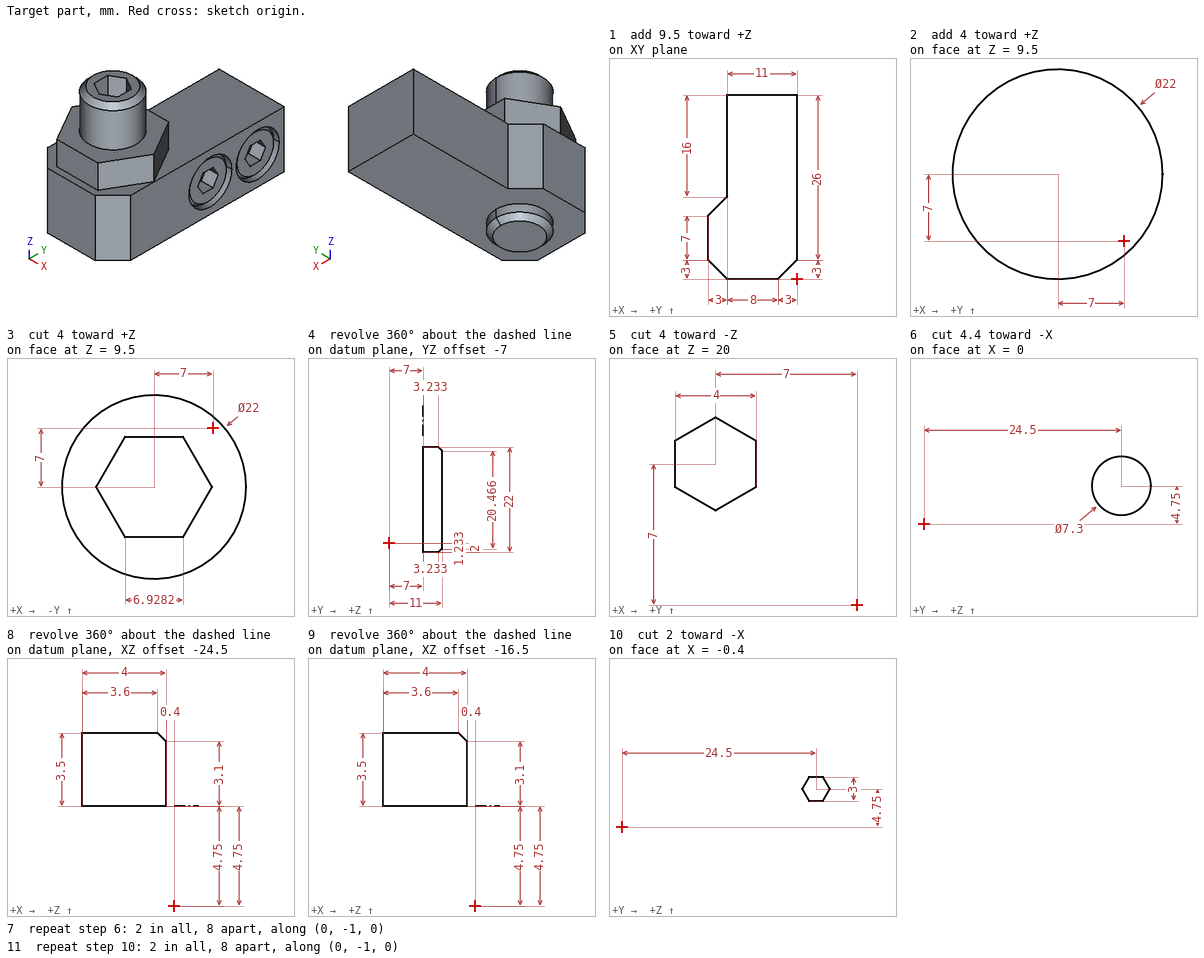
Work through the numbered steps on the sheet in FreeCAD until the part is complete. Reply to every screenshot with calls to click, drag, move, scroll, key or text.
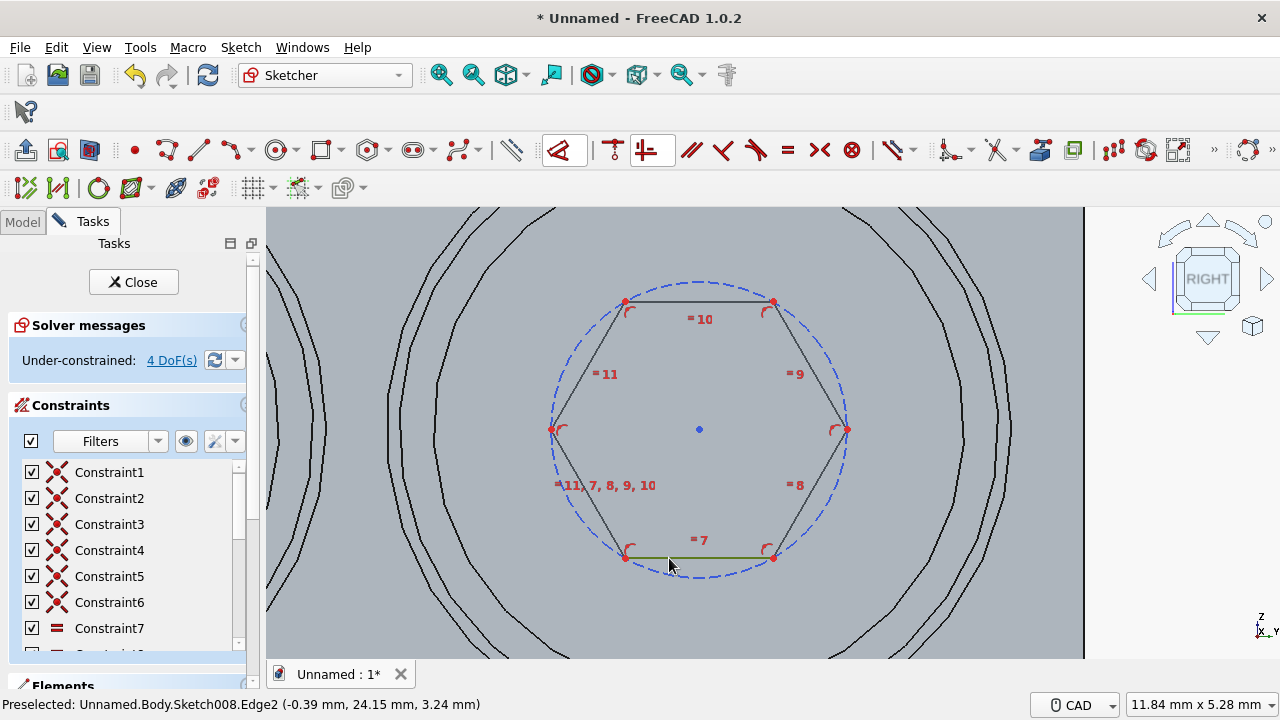
click(670, 150)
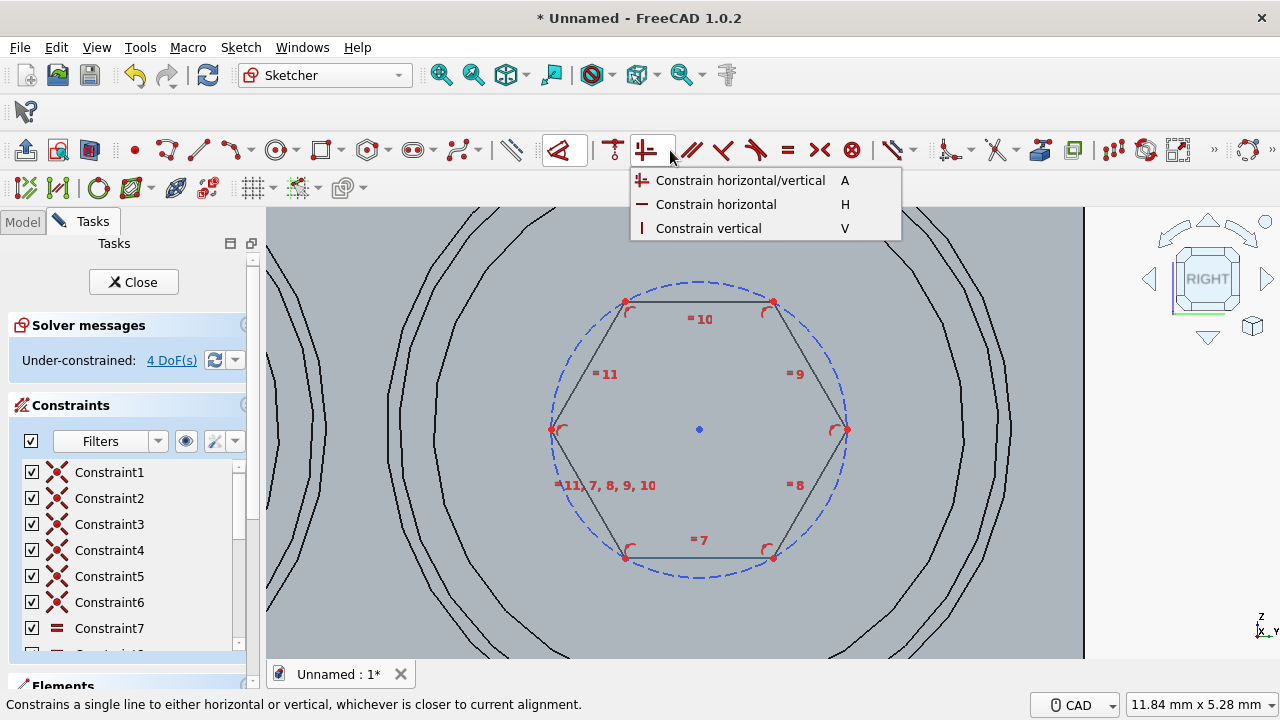
click(766, 204)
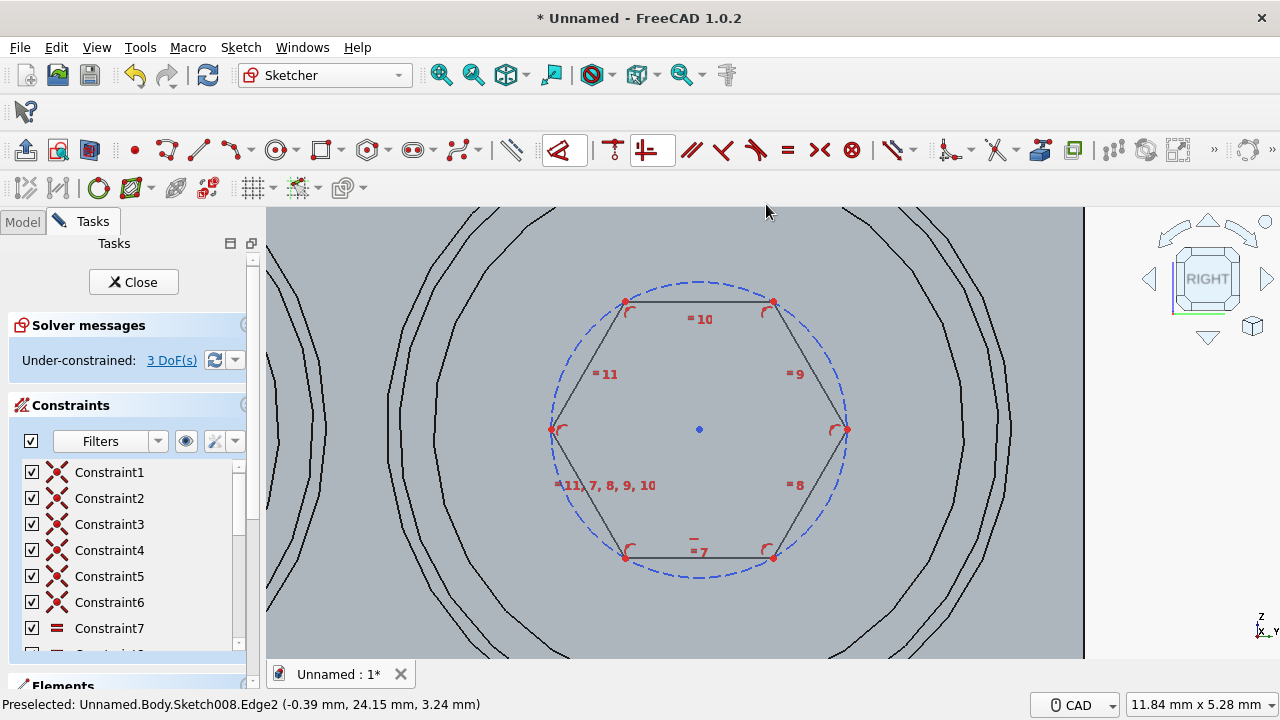
click(625, 558)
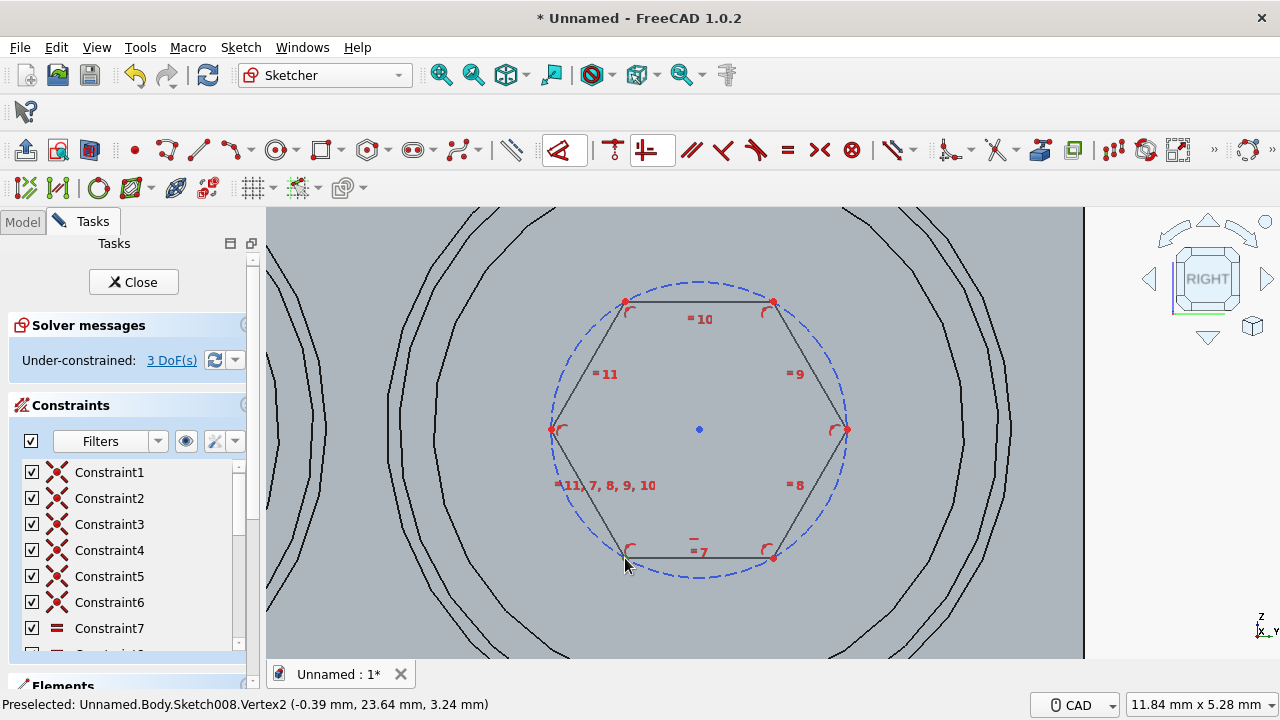
click(773, 302)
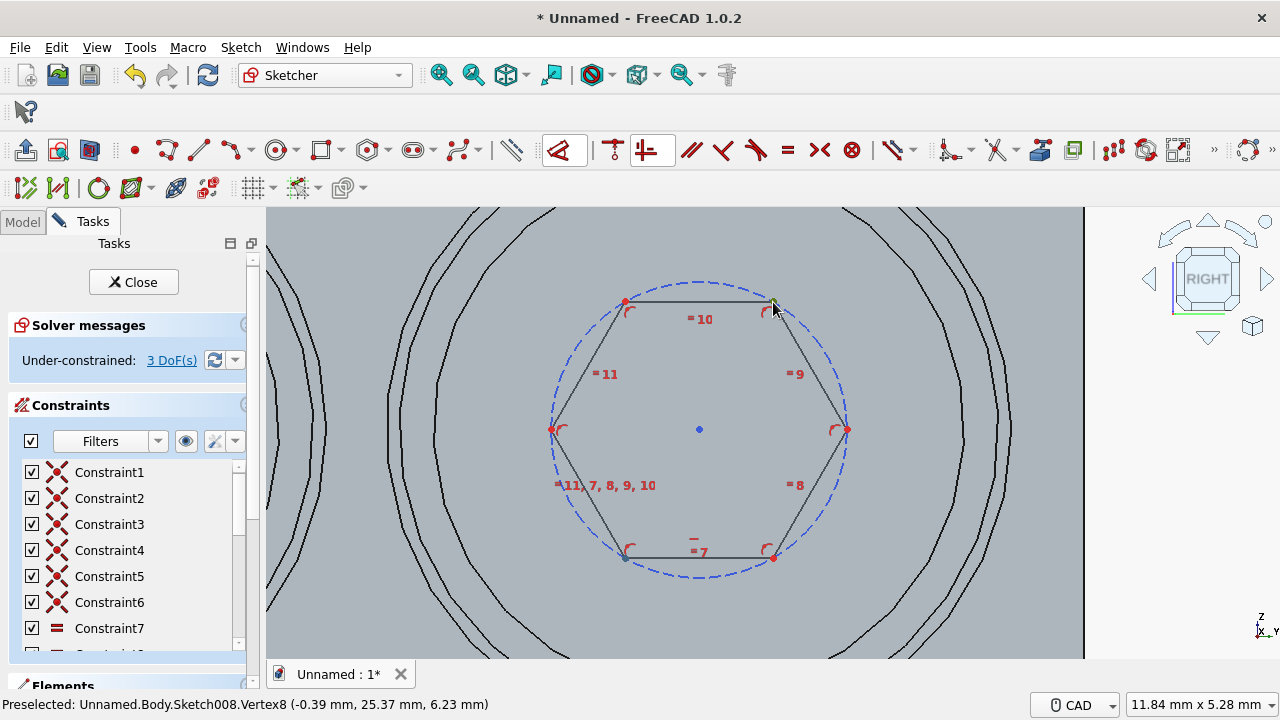
key(i)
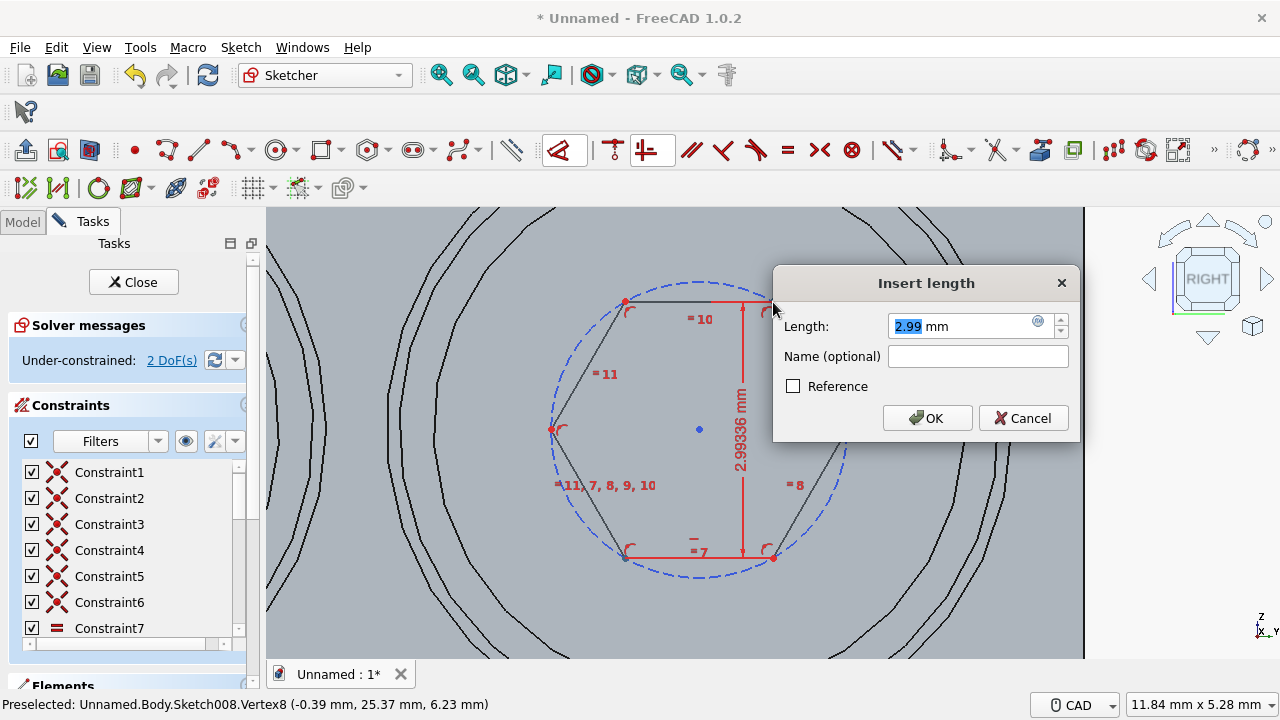
text(3)
key(Return)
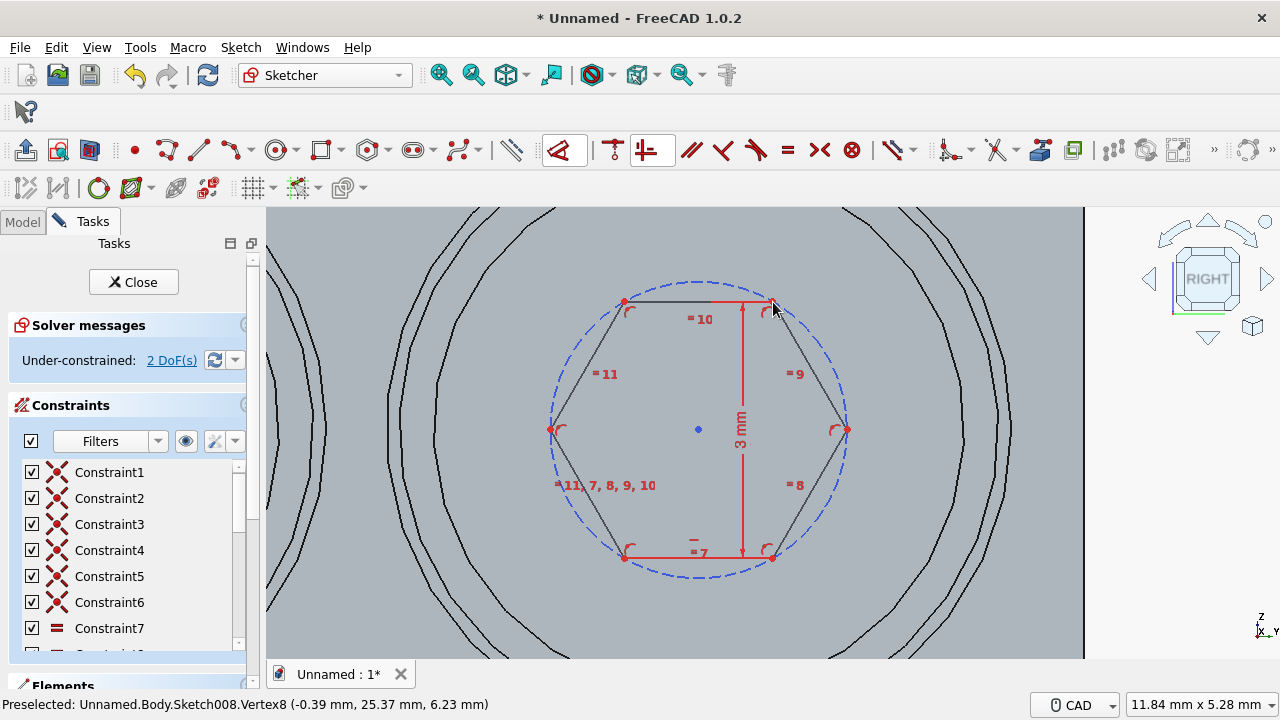
click(699, 430)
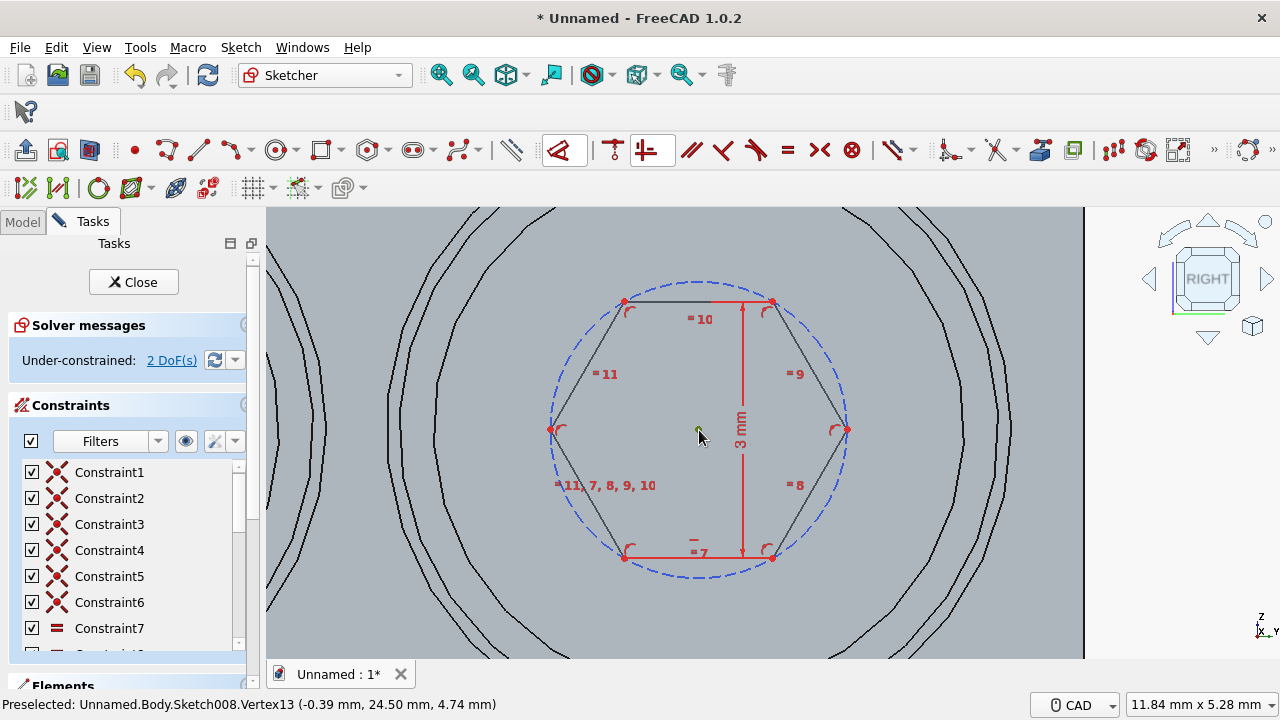
key(l)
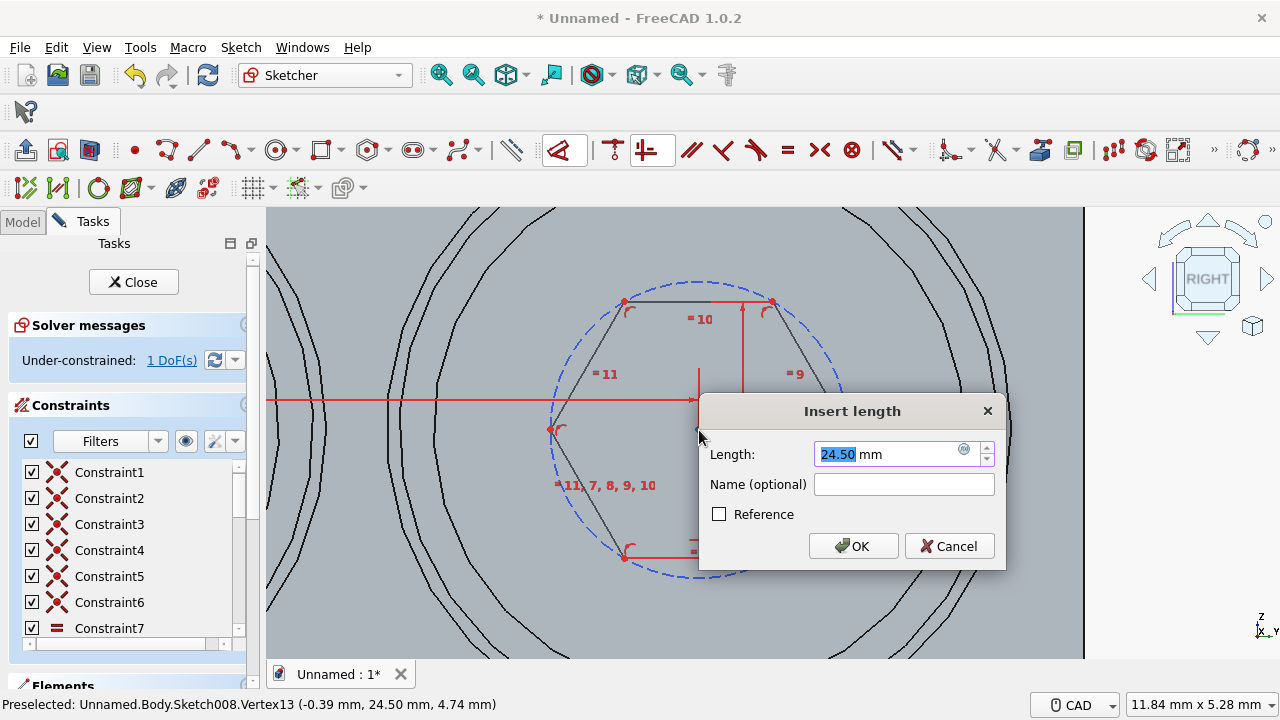
text(24.5)
key(Return)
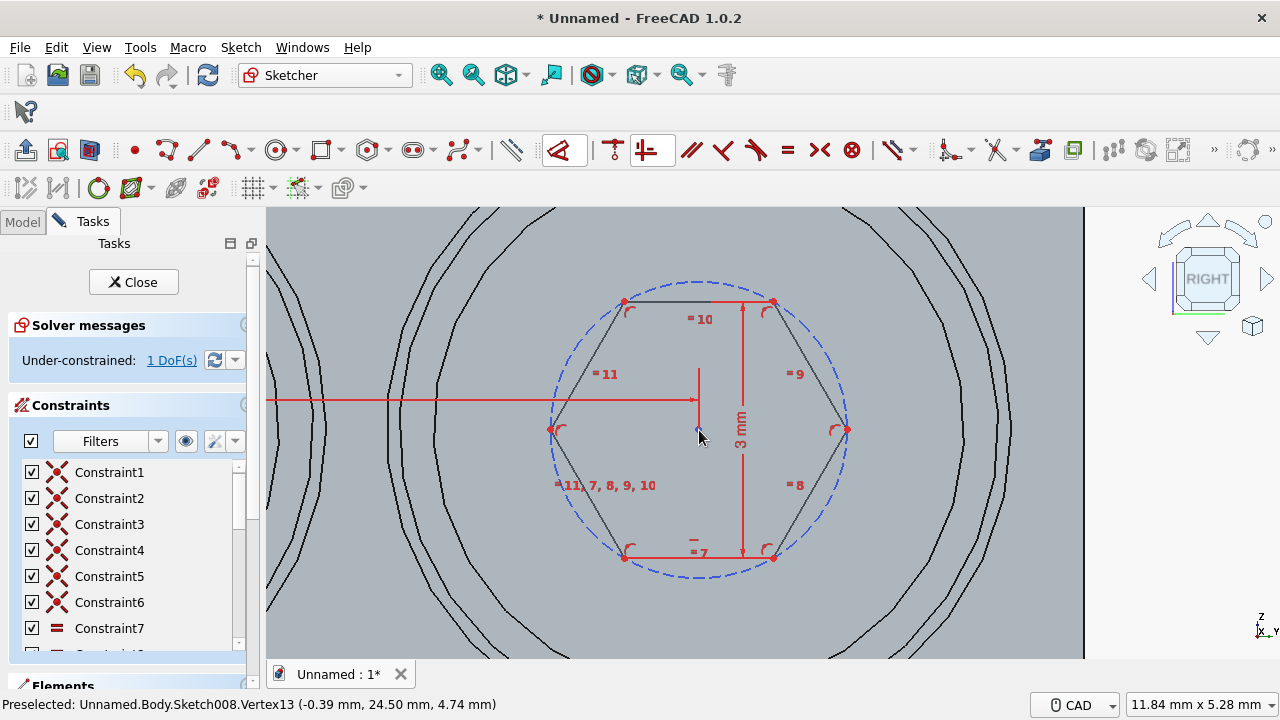
click(699, 430)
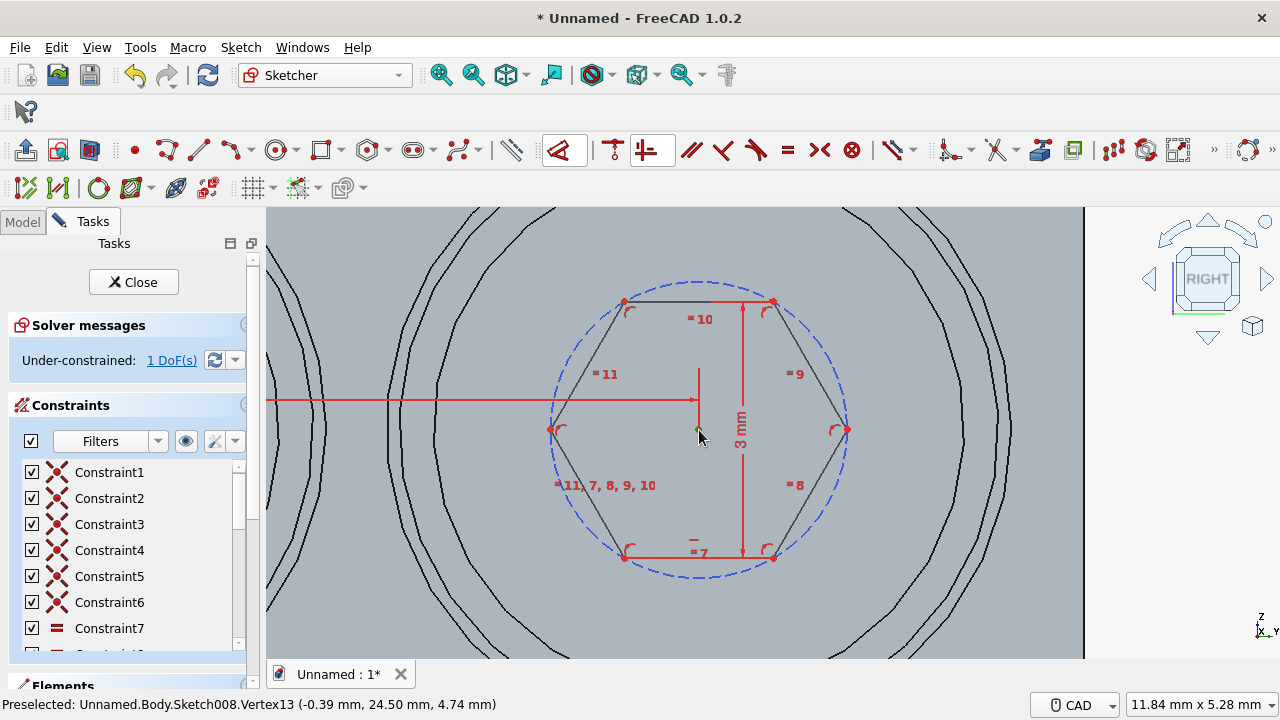
key(i)